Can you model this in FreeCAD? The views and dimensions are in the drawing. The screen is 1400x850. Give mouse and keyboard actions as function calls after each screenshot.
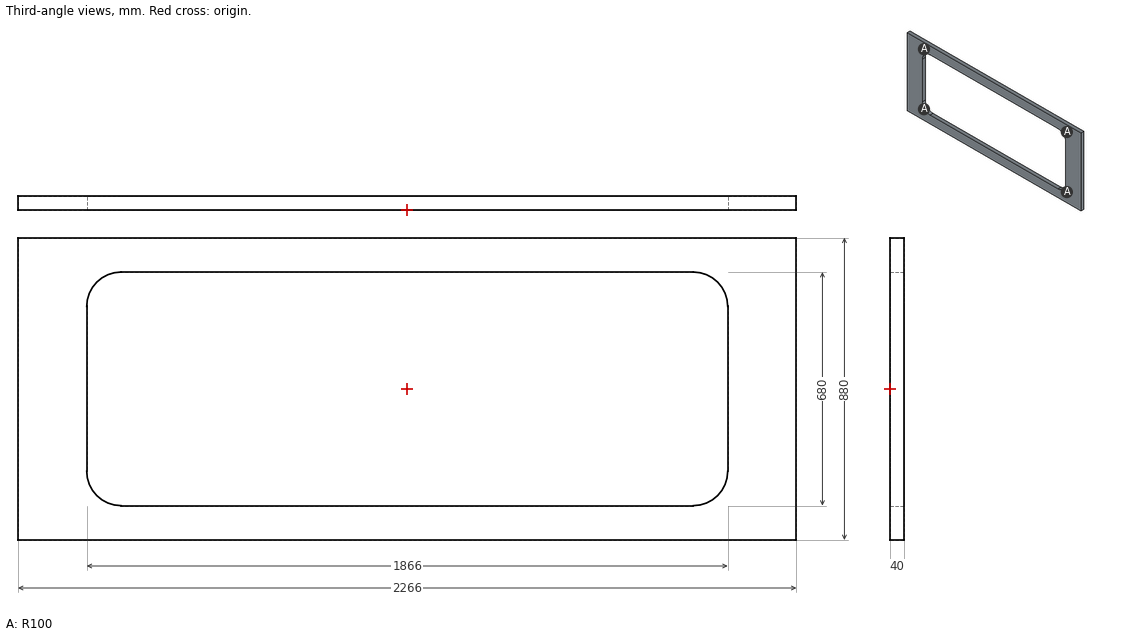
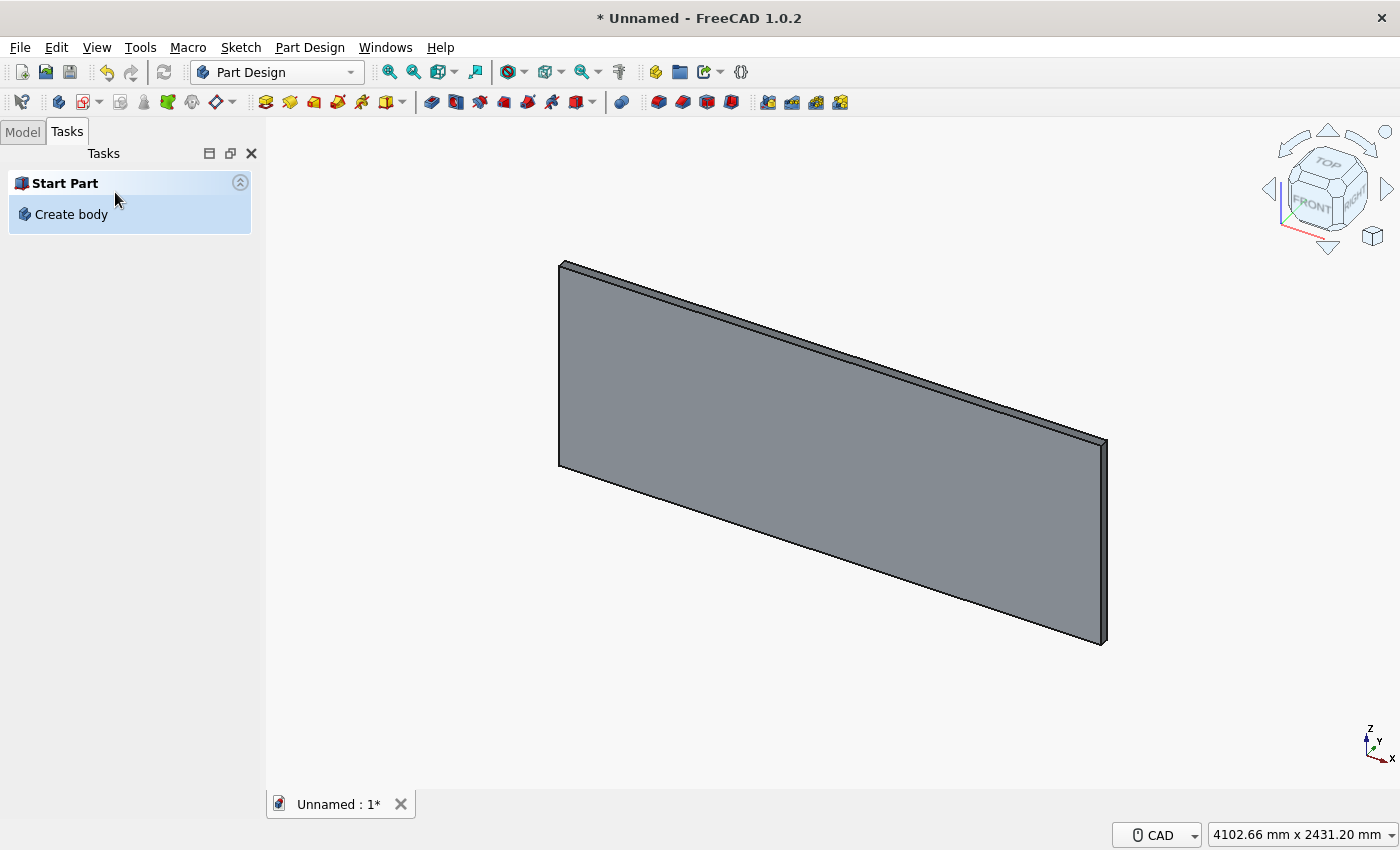
click(985, 506)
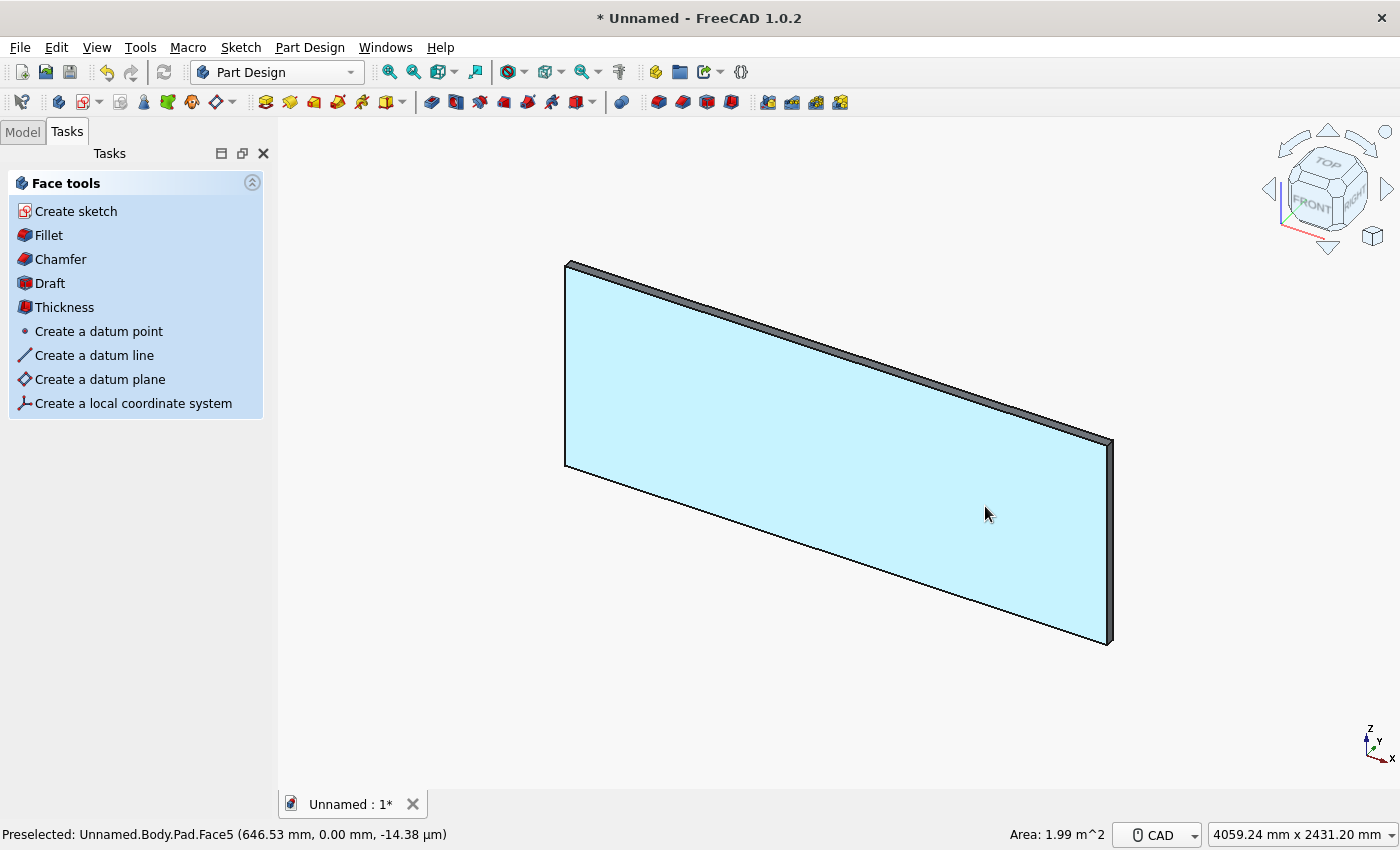
click(84, 102)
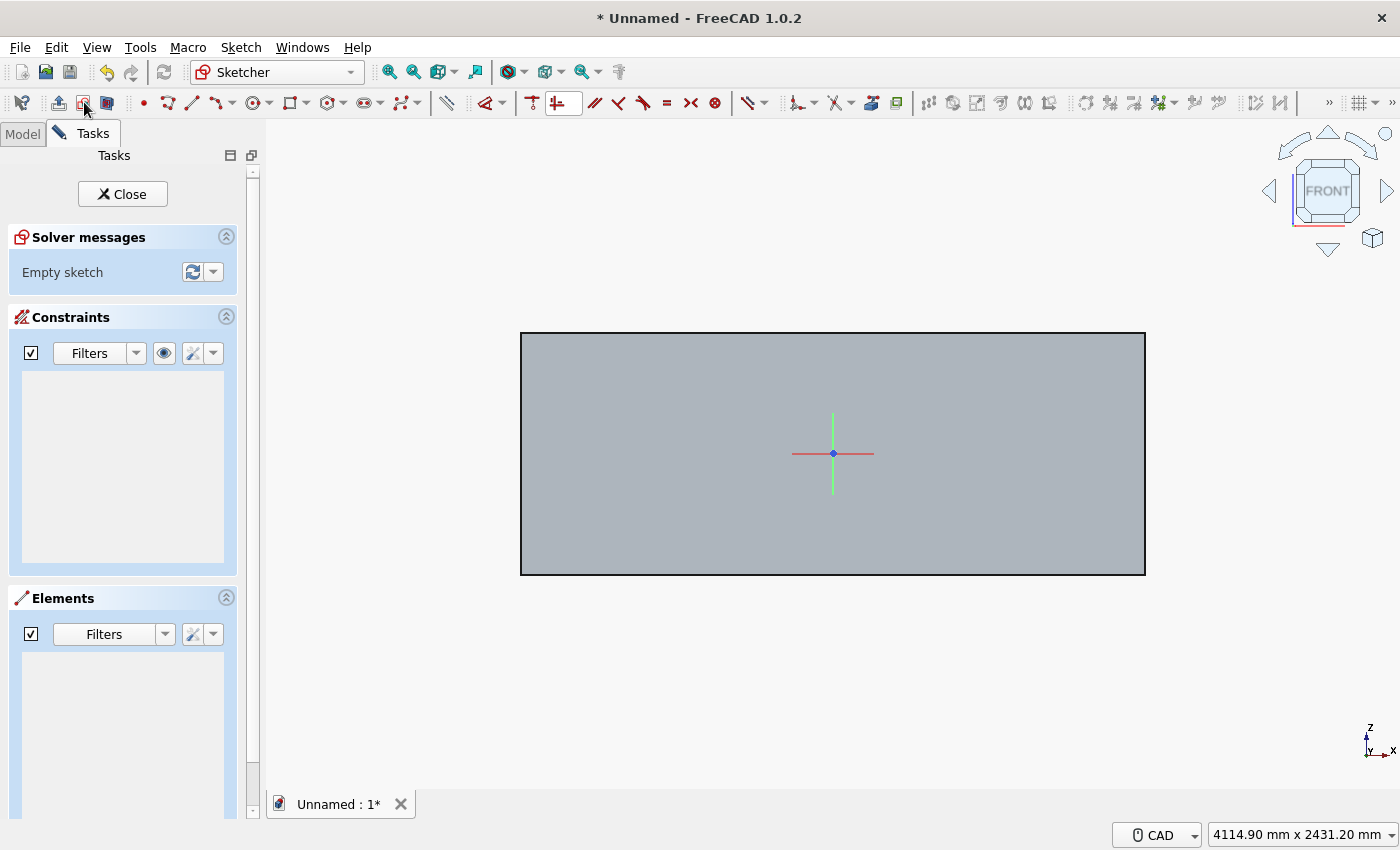
key(g)
key(v)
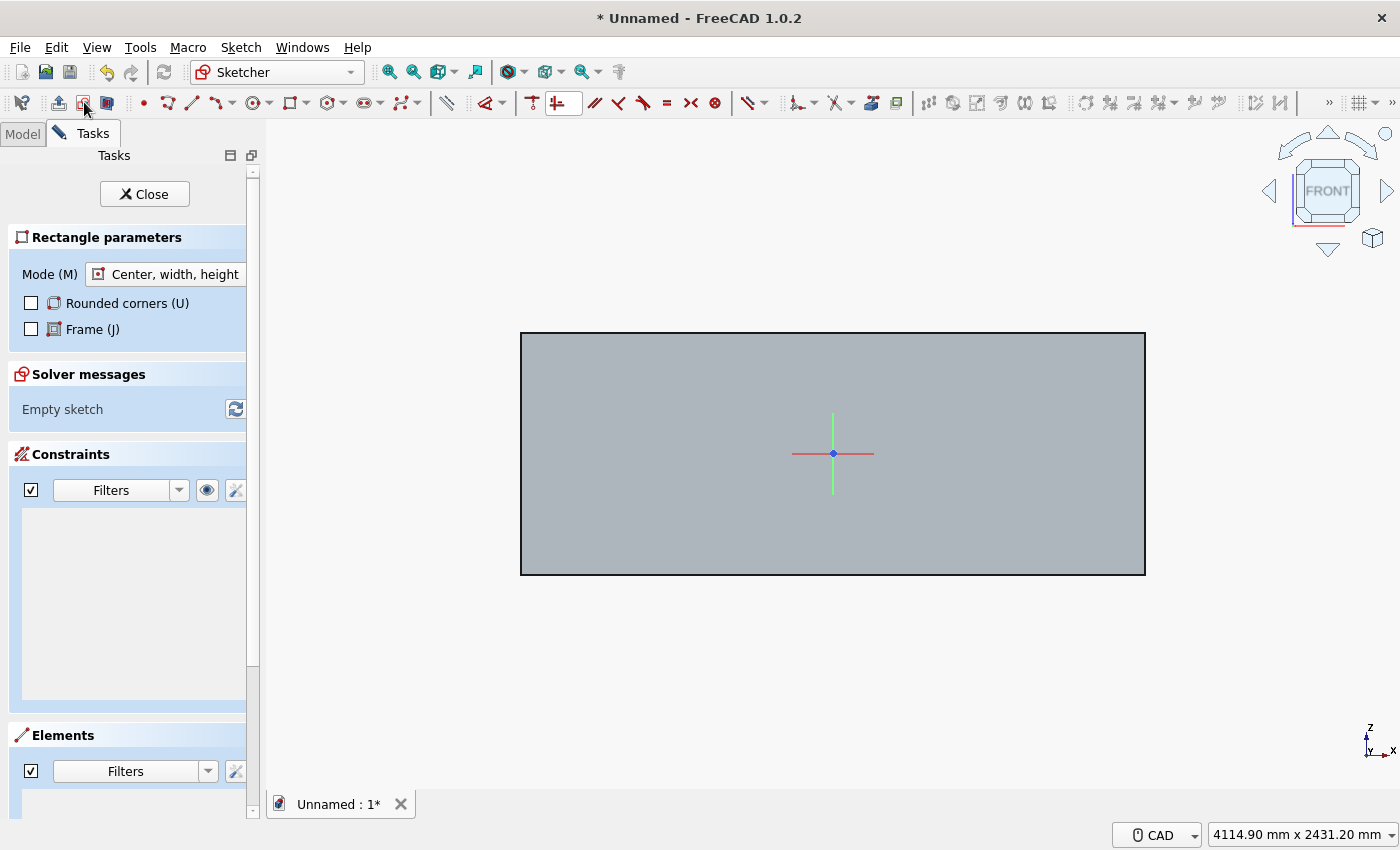
click(833, 454)
click(1090, 360)
key(Escape)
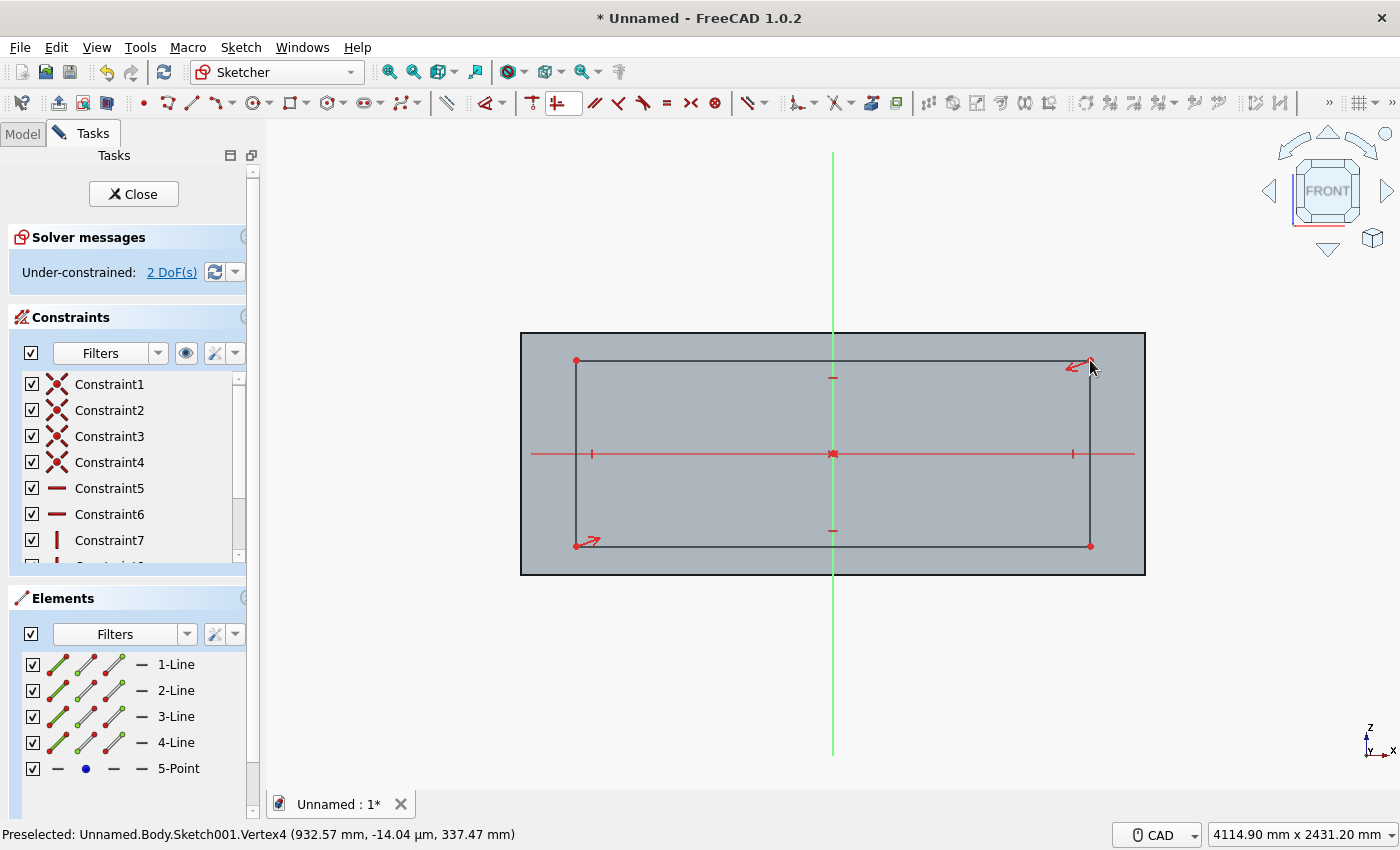
key(d)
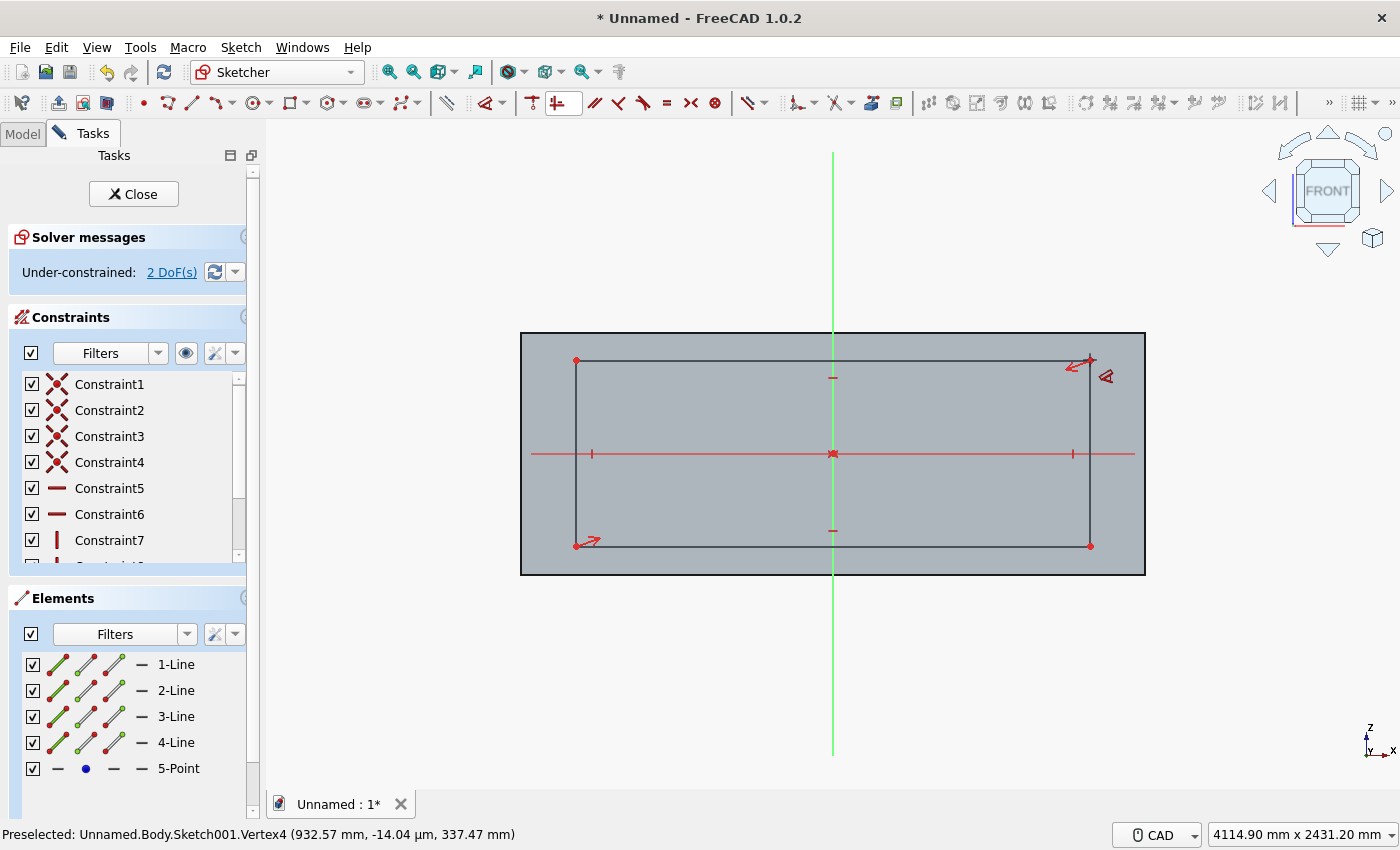
click(1090, 491)
click(1124, 411)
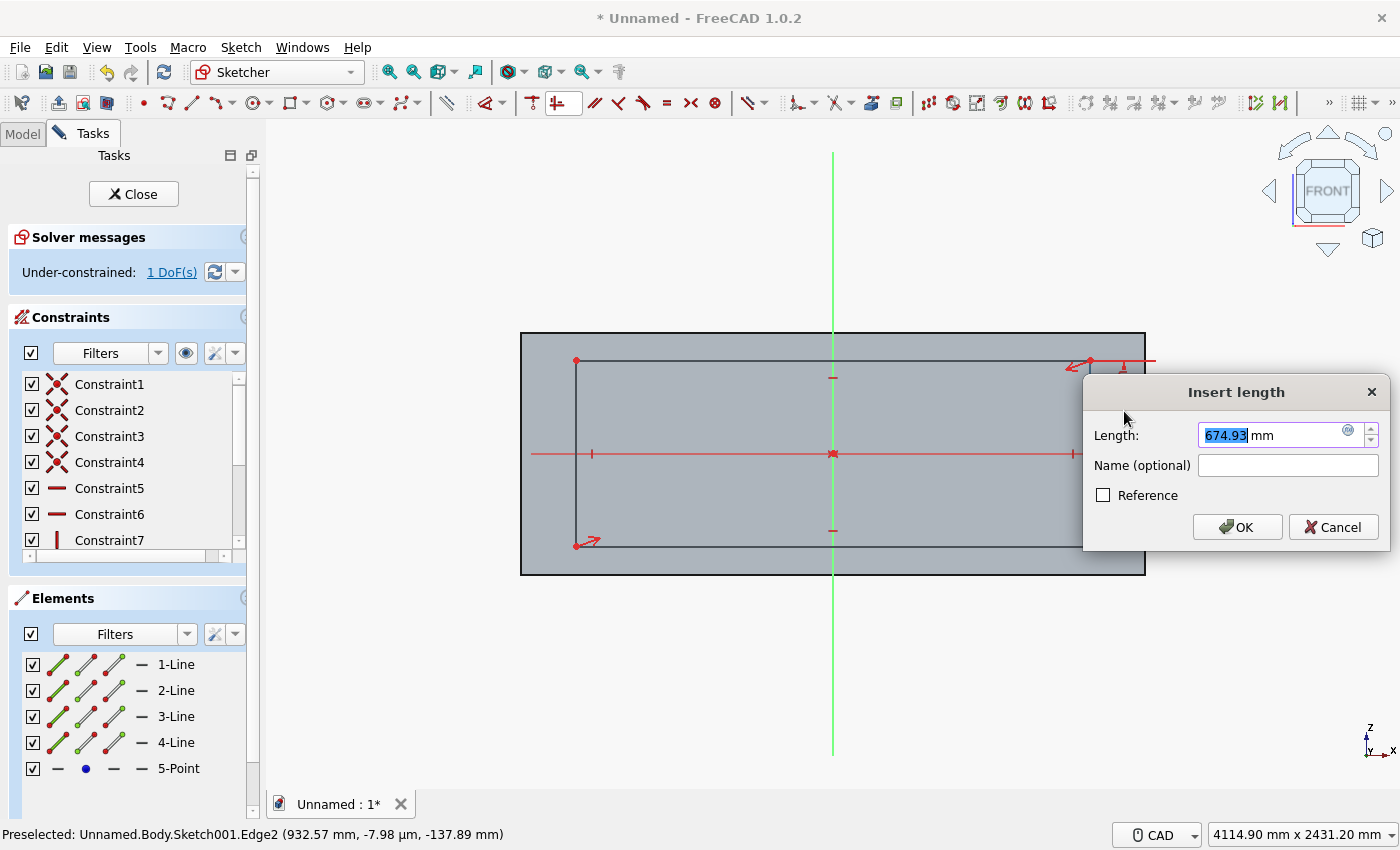
text(680)
key(Return)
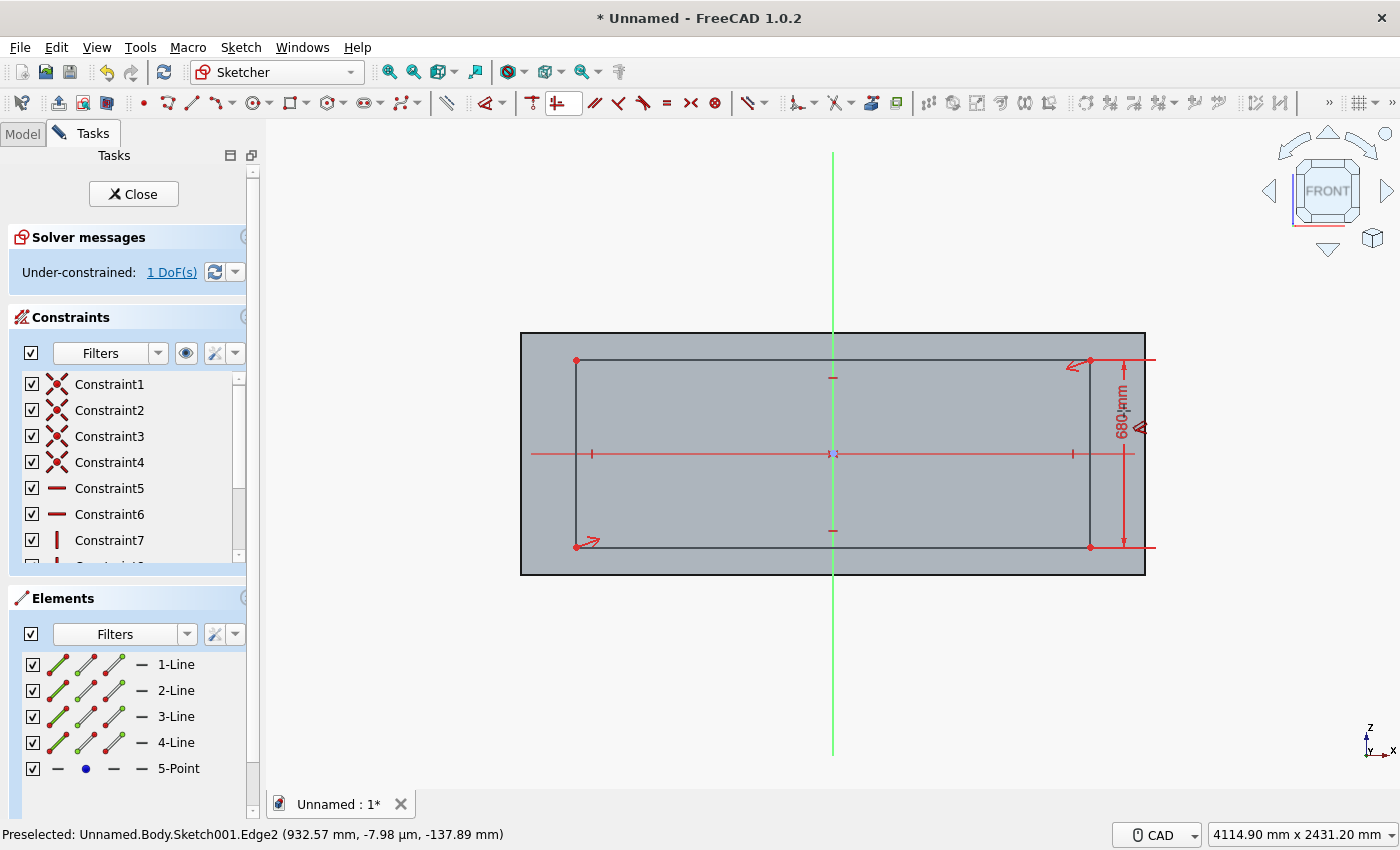
click(730, 548)
click(715, 582)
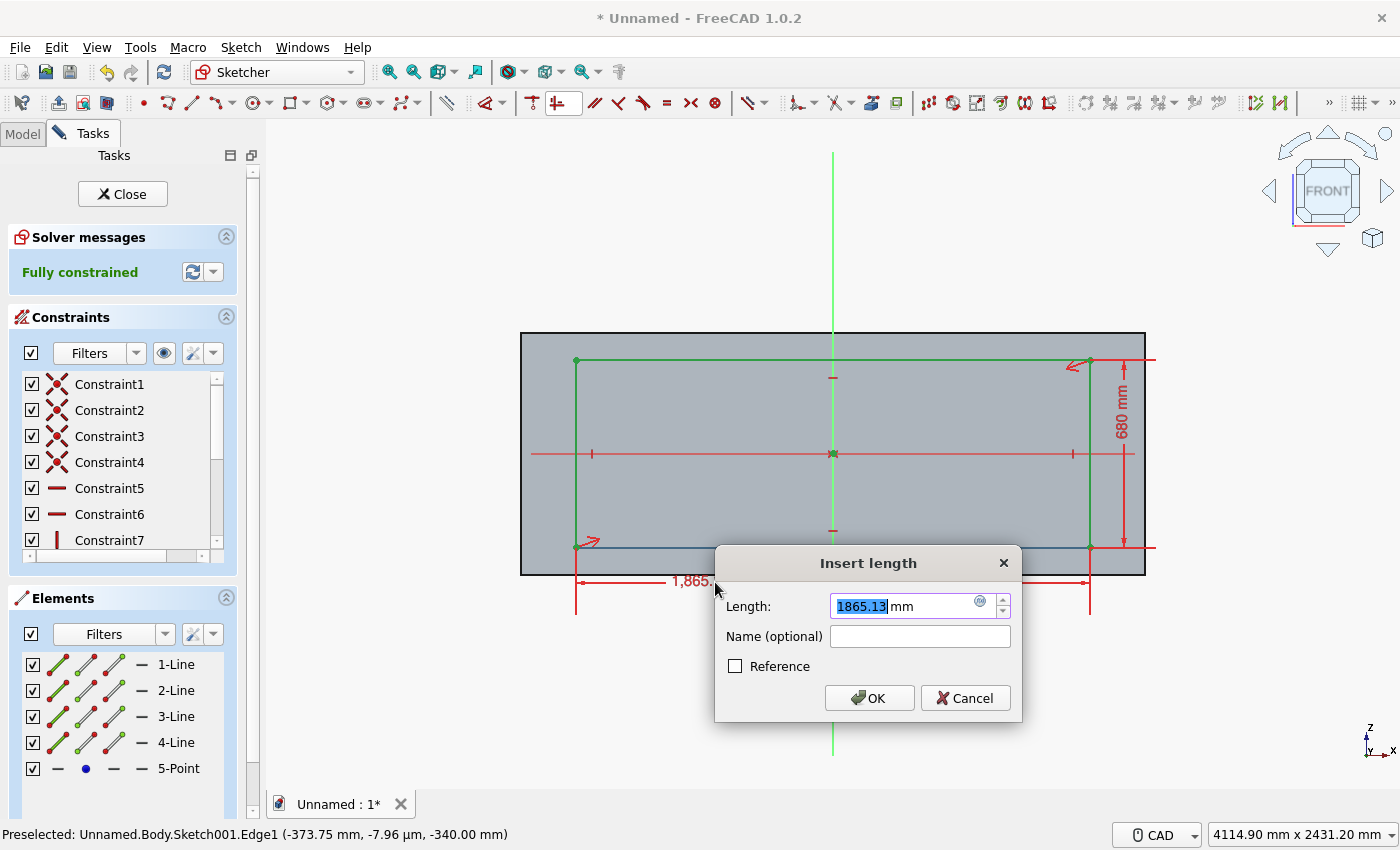
text(1866)
key(Return)
key(Escape)